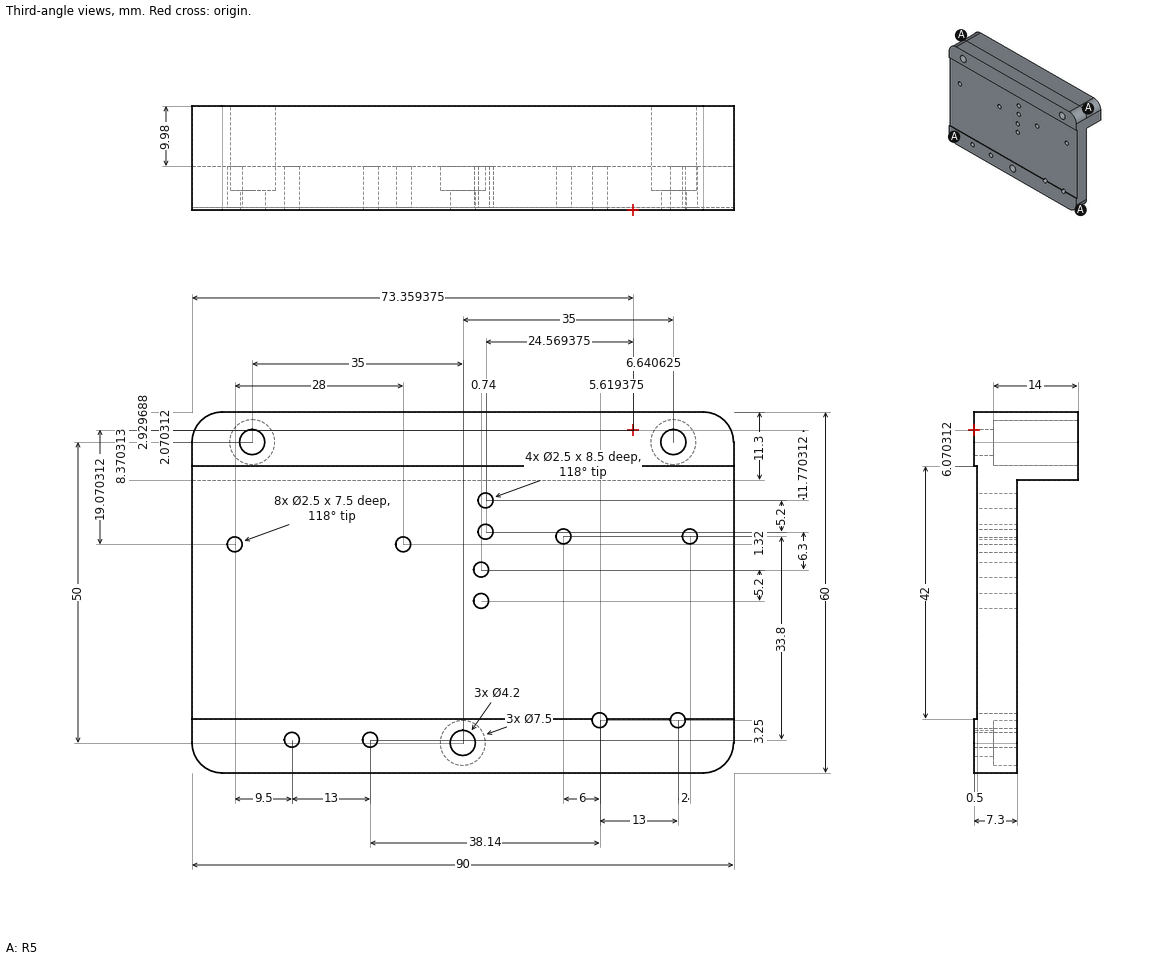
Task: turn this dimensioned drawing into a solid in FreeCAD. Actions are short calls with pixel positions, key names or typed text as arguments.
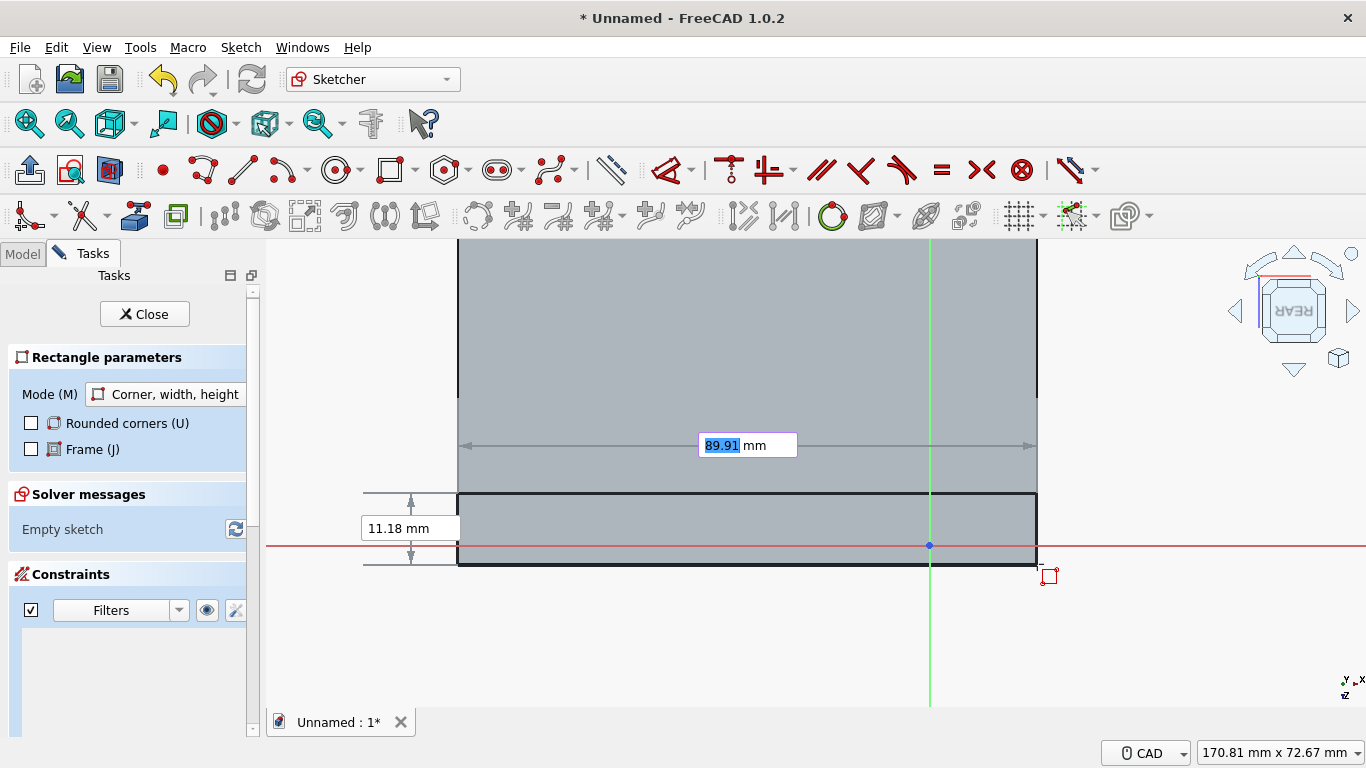
text(90)
key(Tab)
text(11.3)
key(Return)
key(Escape)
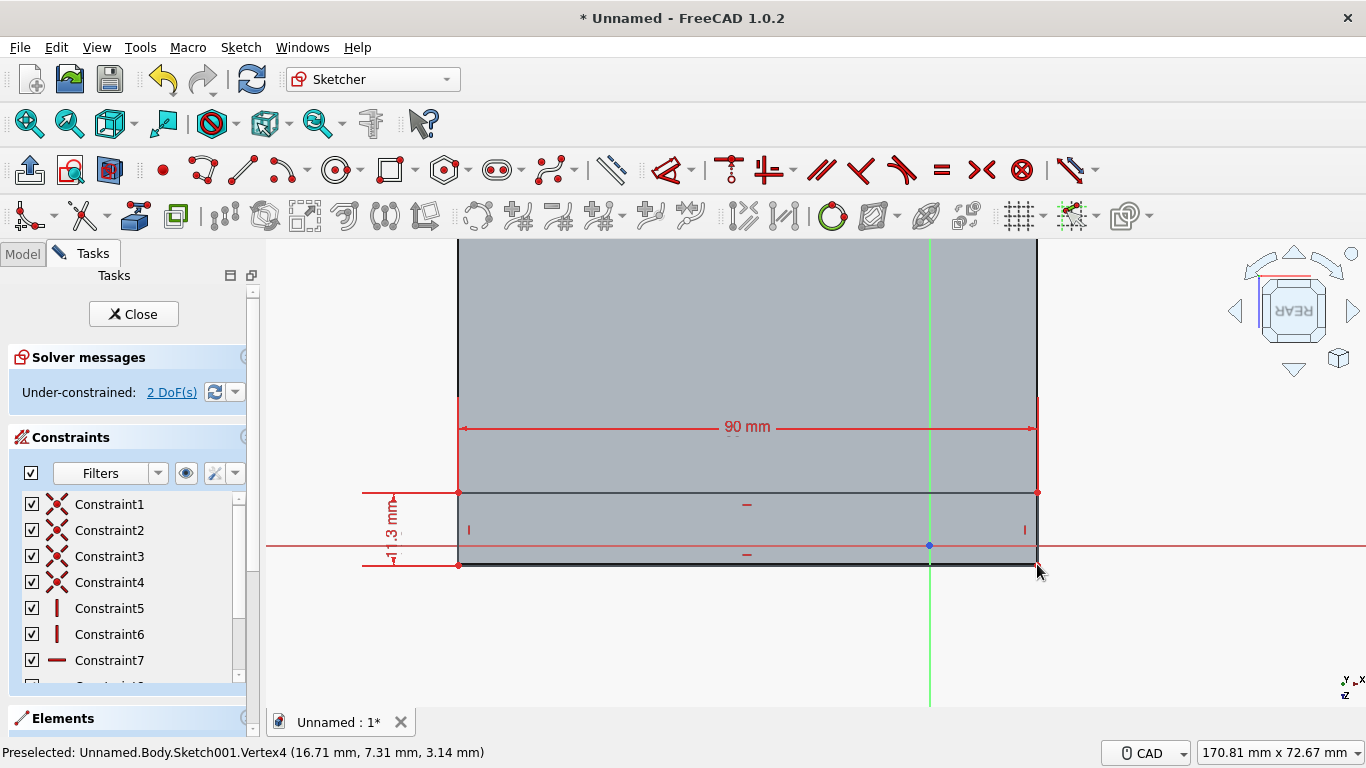
click(666, 170)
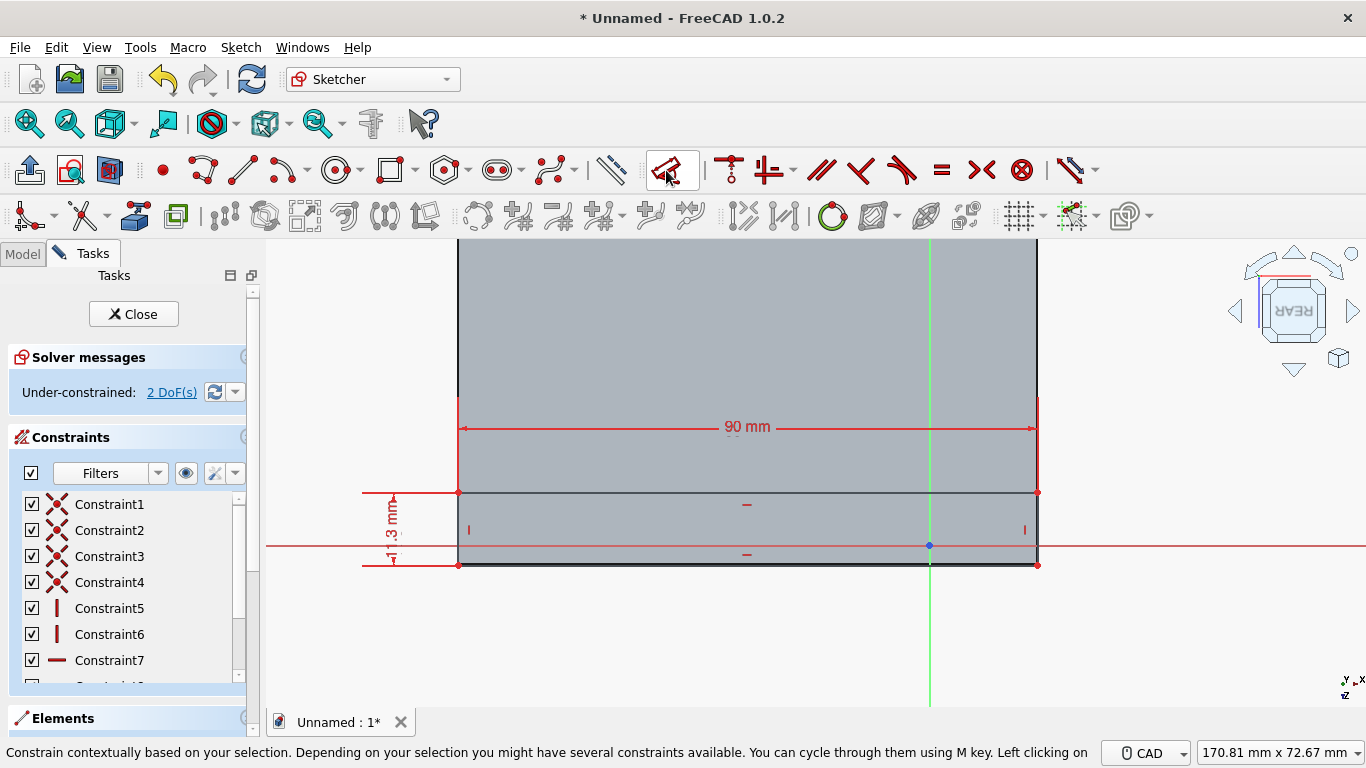
click(458, 493)
click(424, 519)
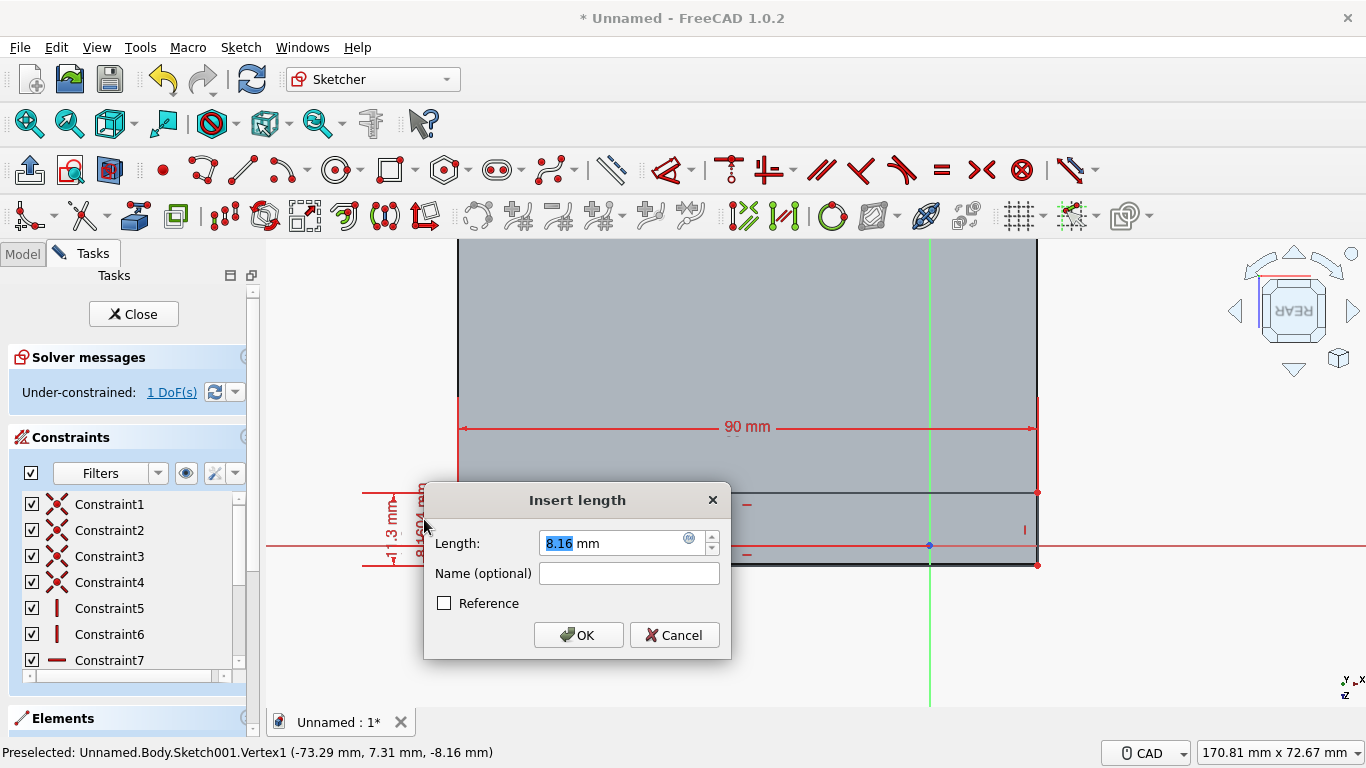
text(8.370313)
key(Return)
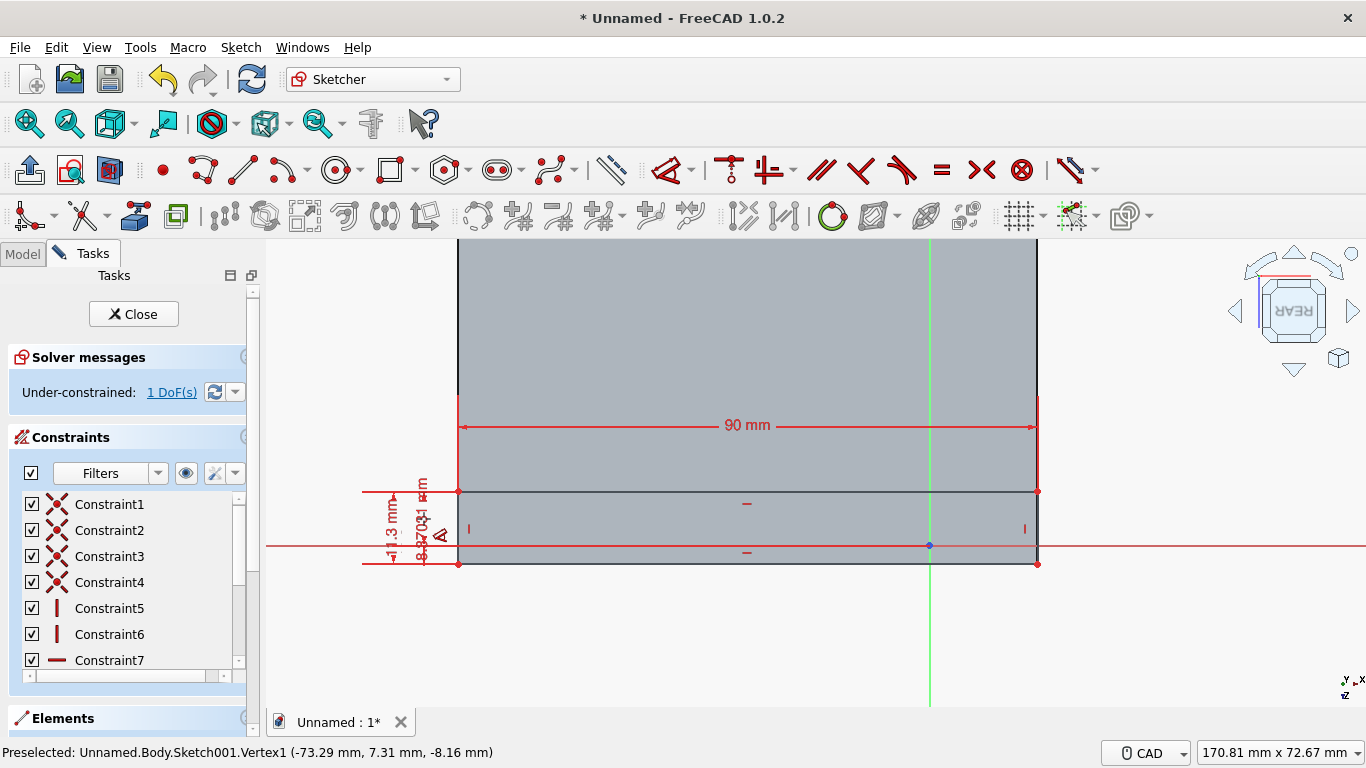
click(458, 492)
click(694, 458)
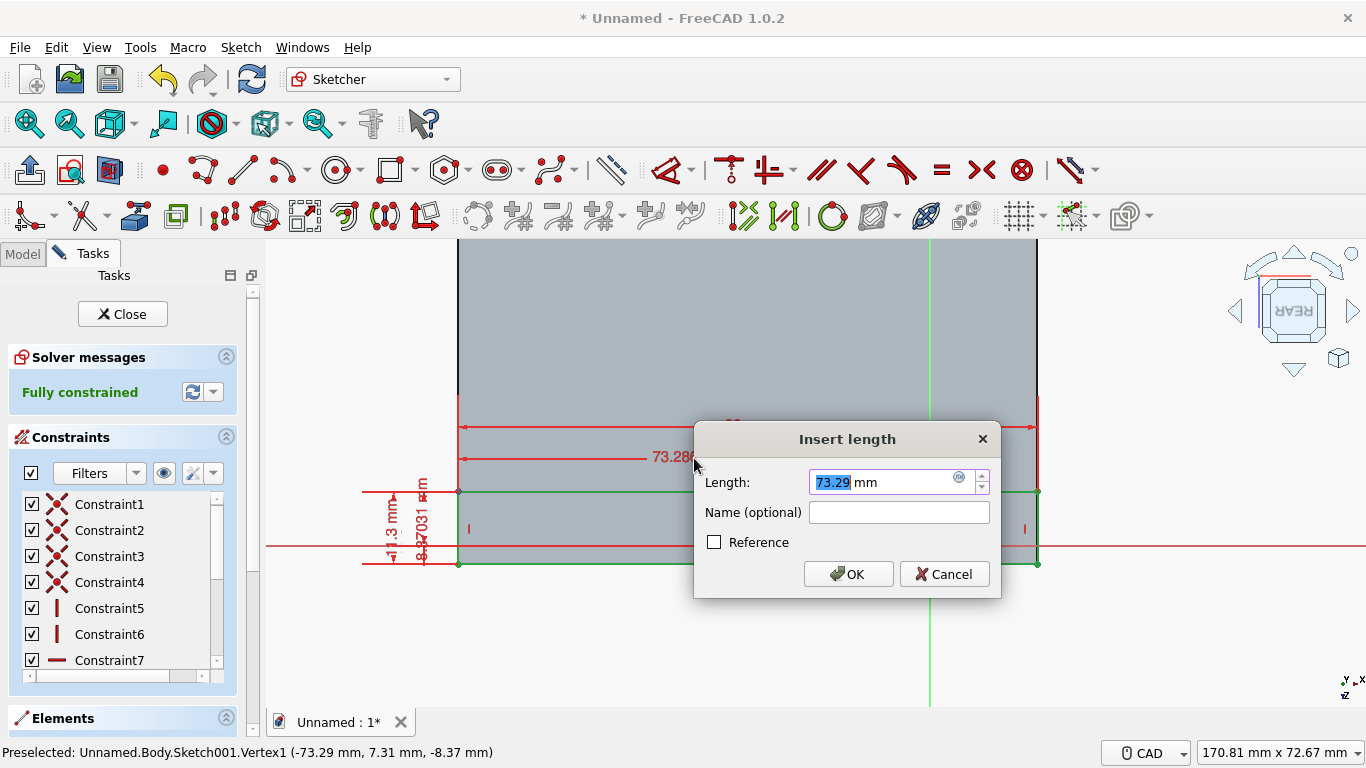
text(73.359375)
key(Return)
key(Escape)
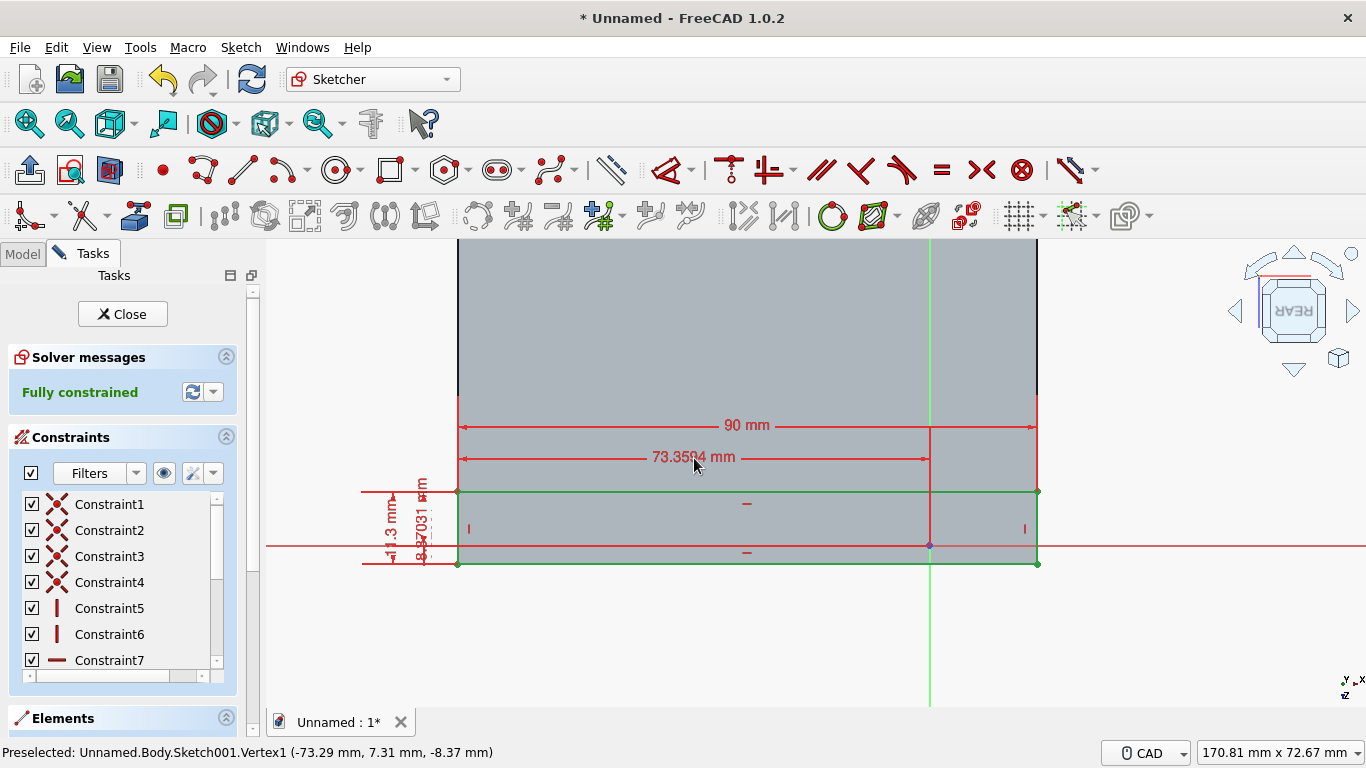
click(123, 314)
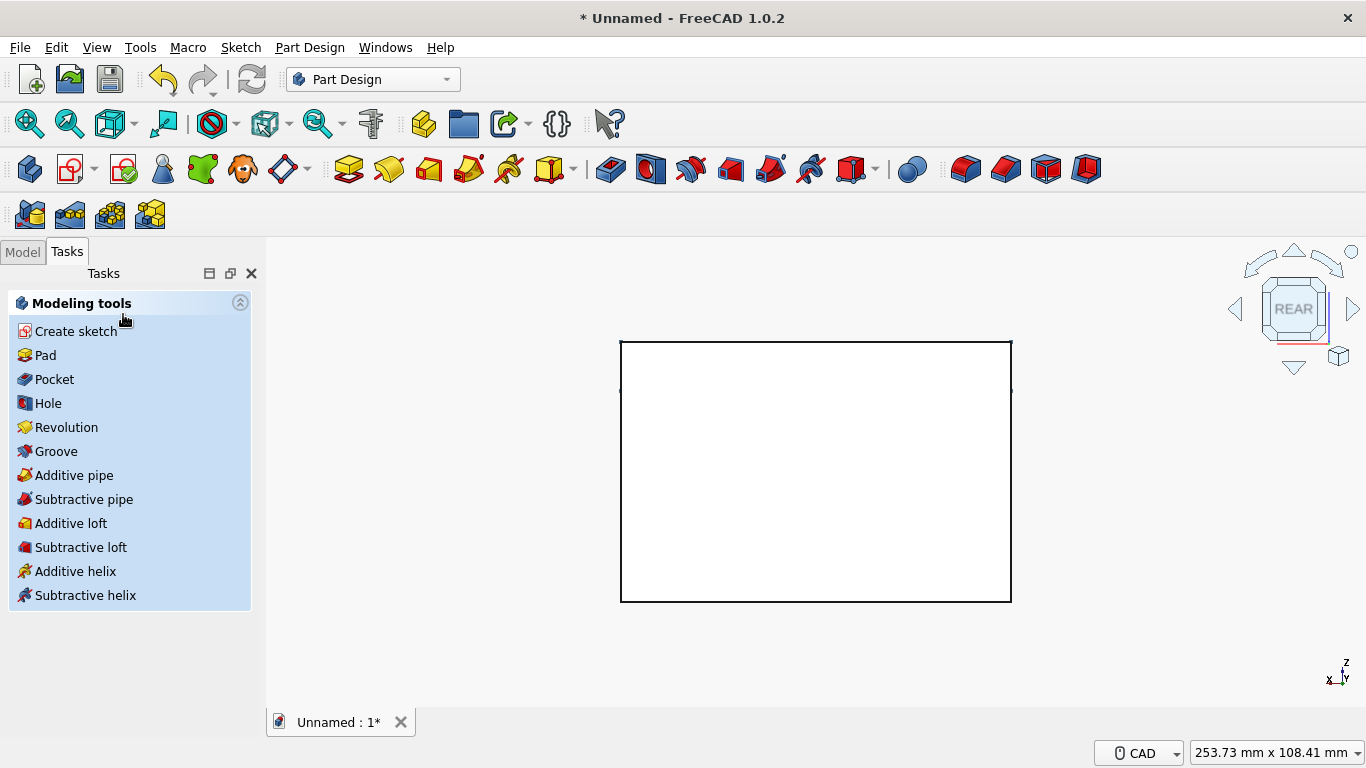
click(350, 170)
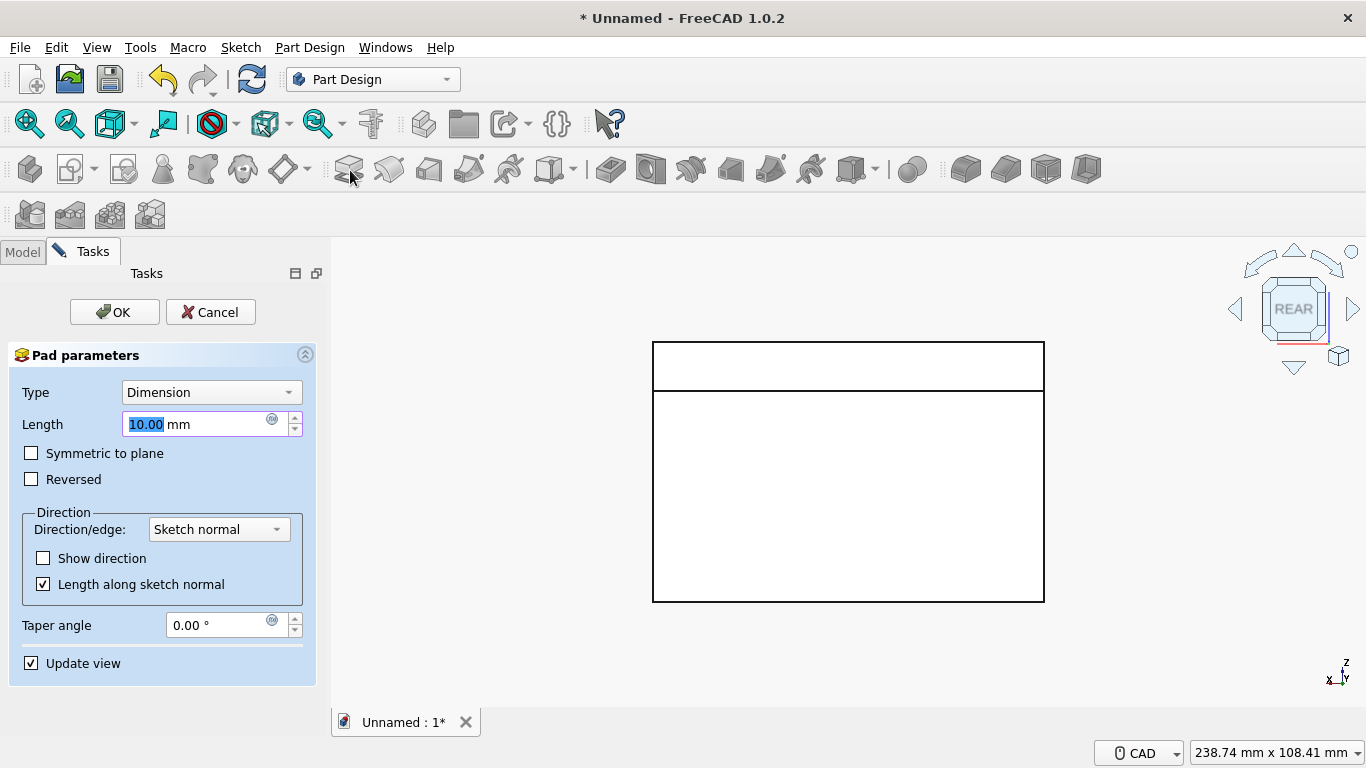
text(9.98)
key(Tab)